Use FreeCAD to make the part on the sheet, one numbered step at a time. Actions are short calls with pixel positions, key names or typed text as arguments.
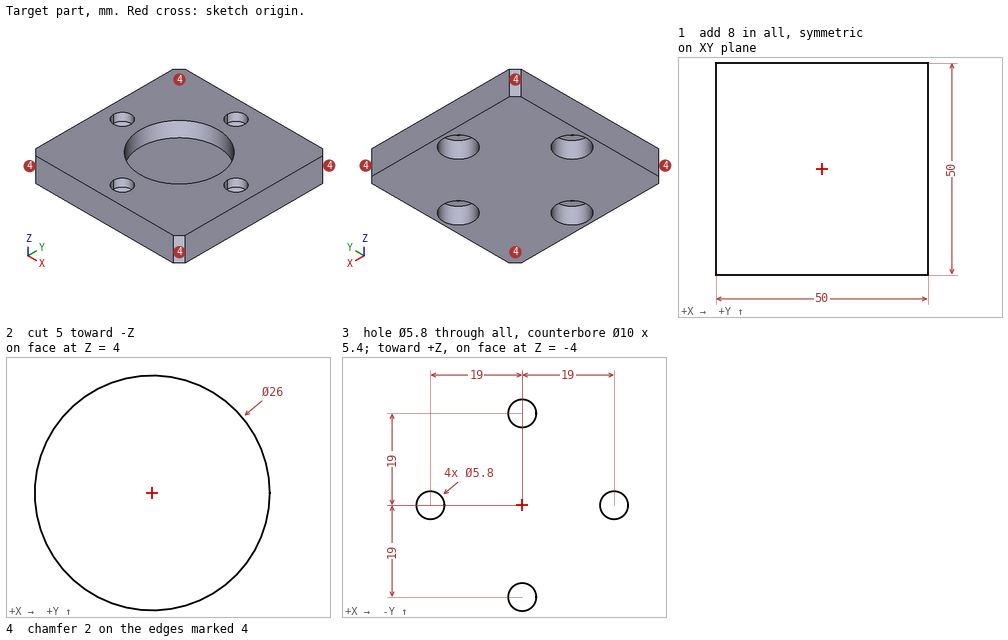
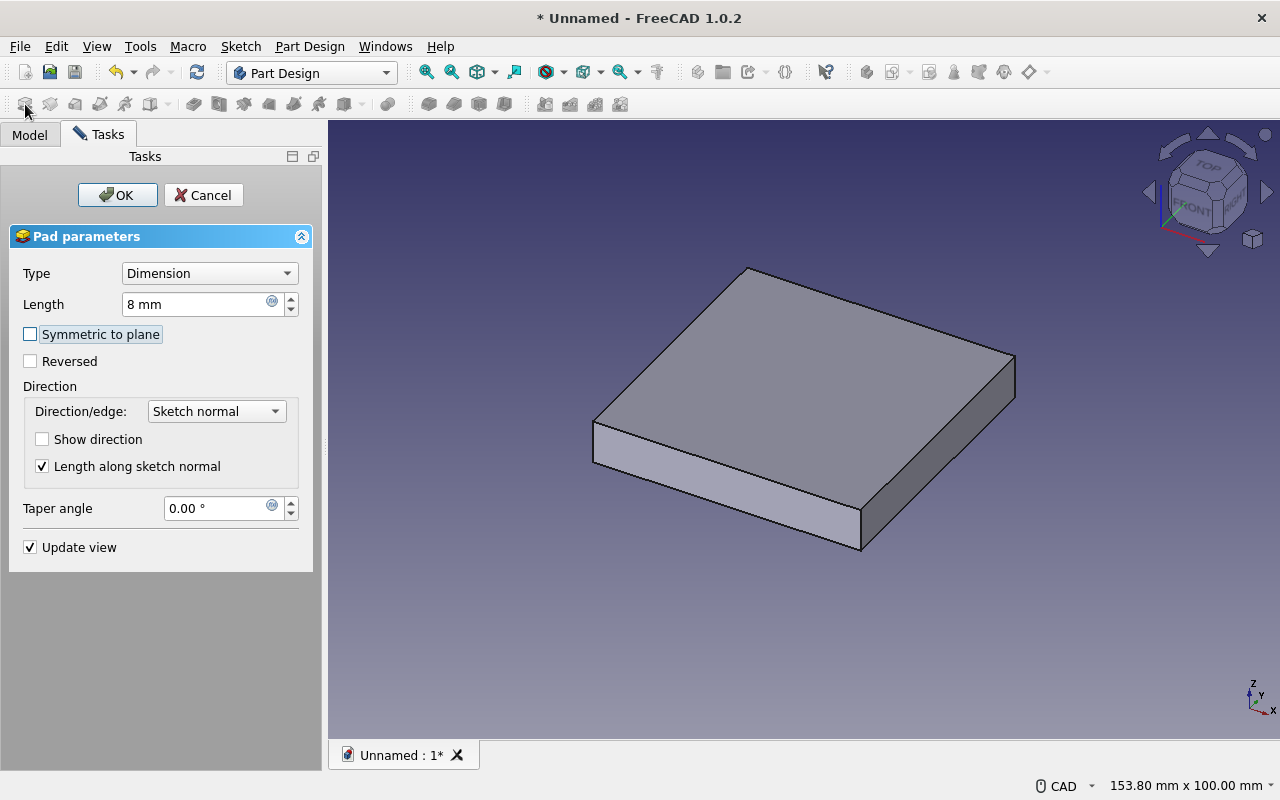
click(31, 334)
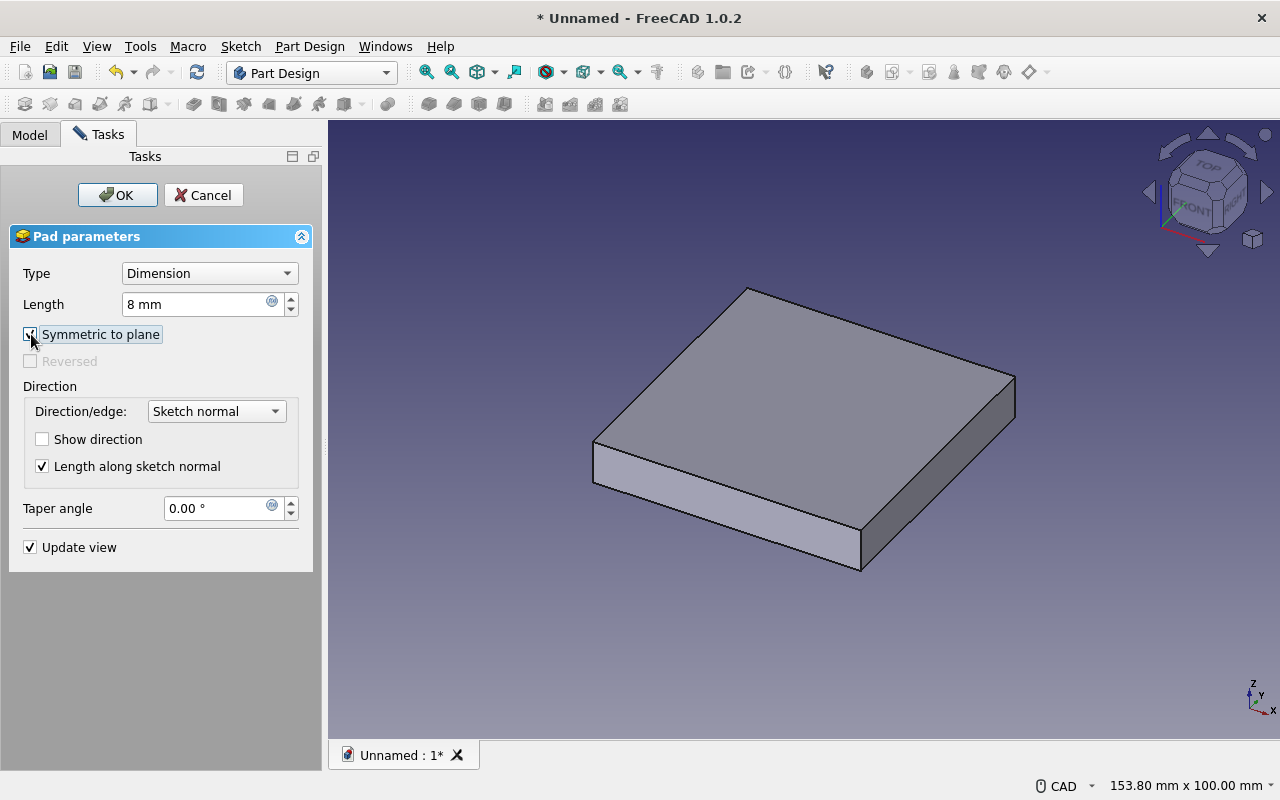
click(118, 195)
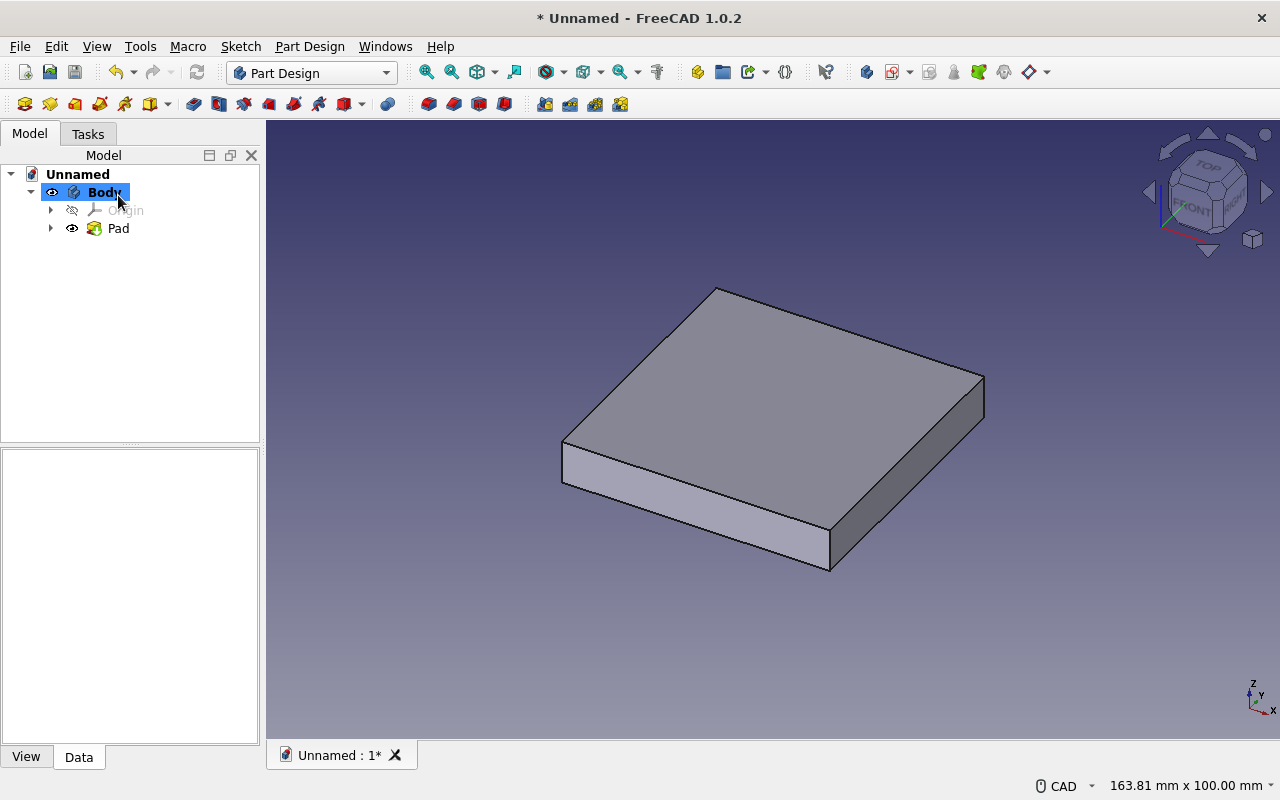
click(773, 408)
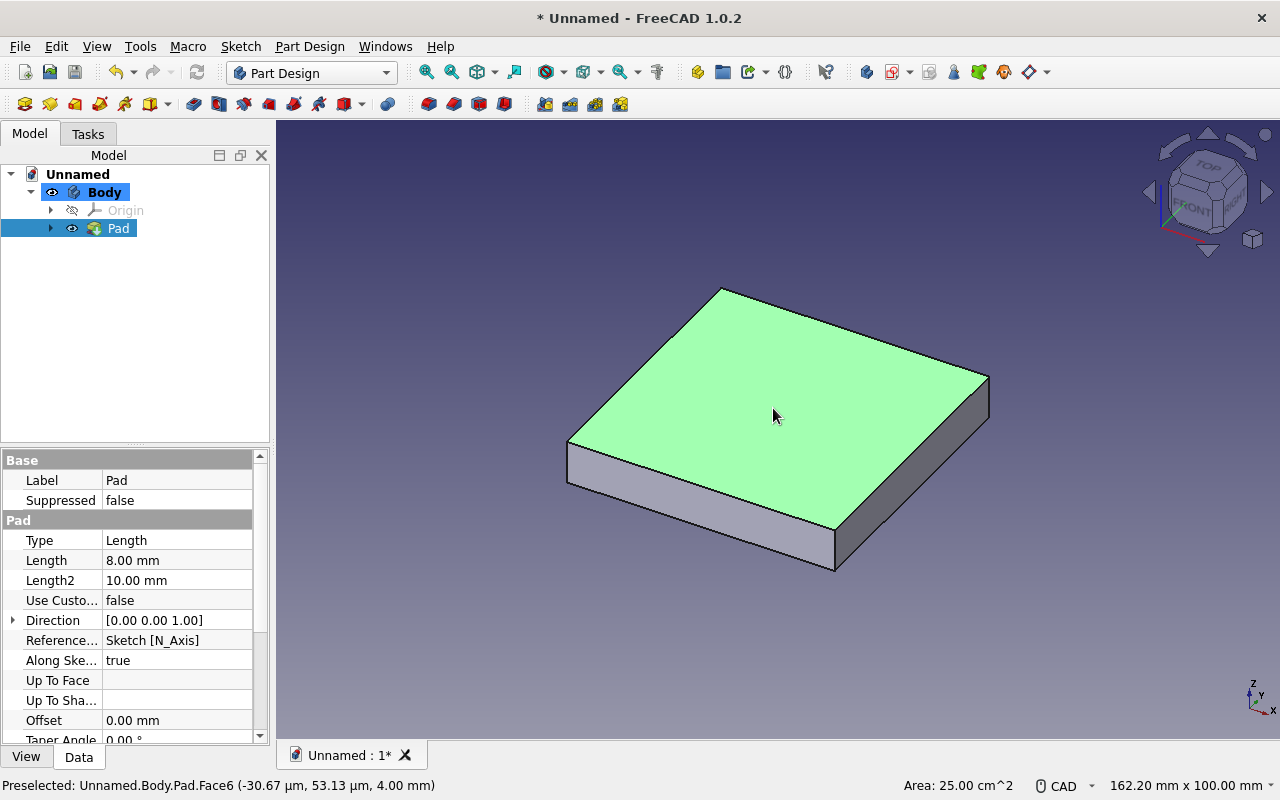
click(892, 72)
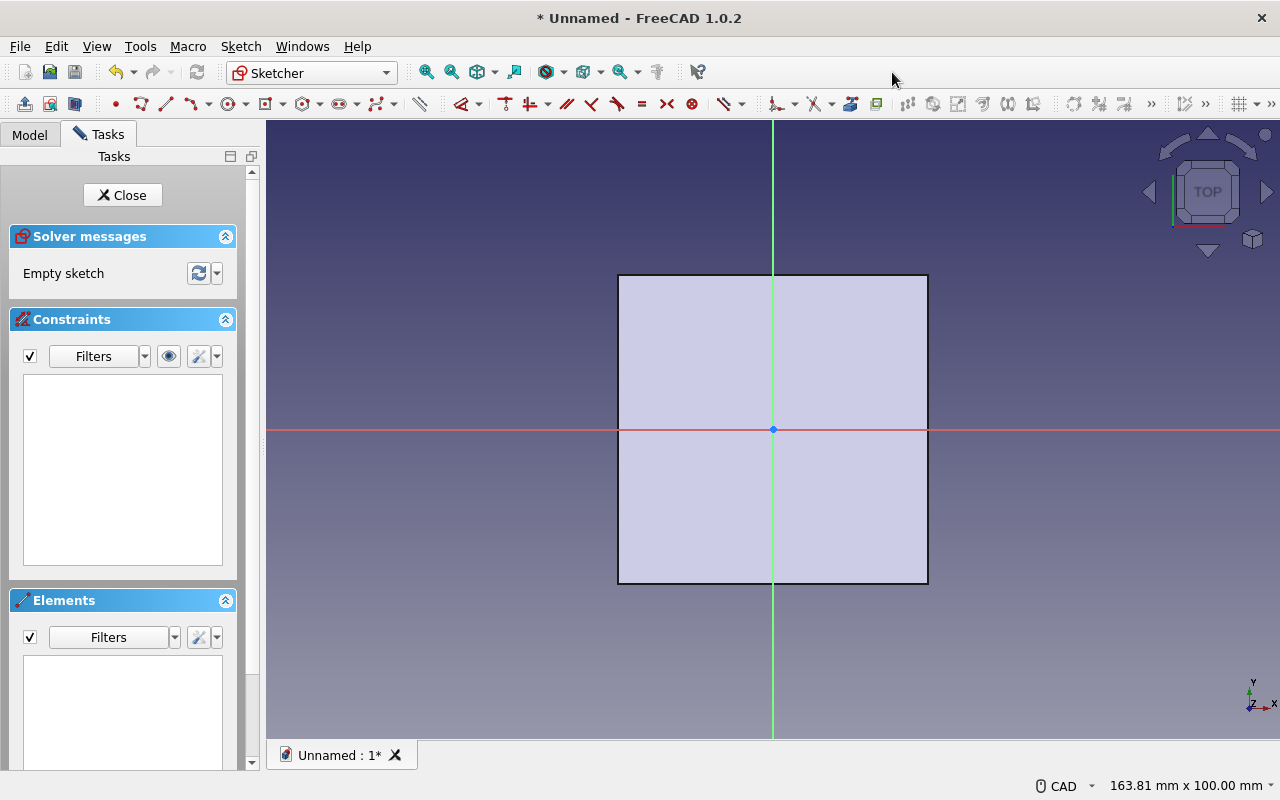
scroll(813, 429, up, 5)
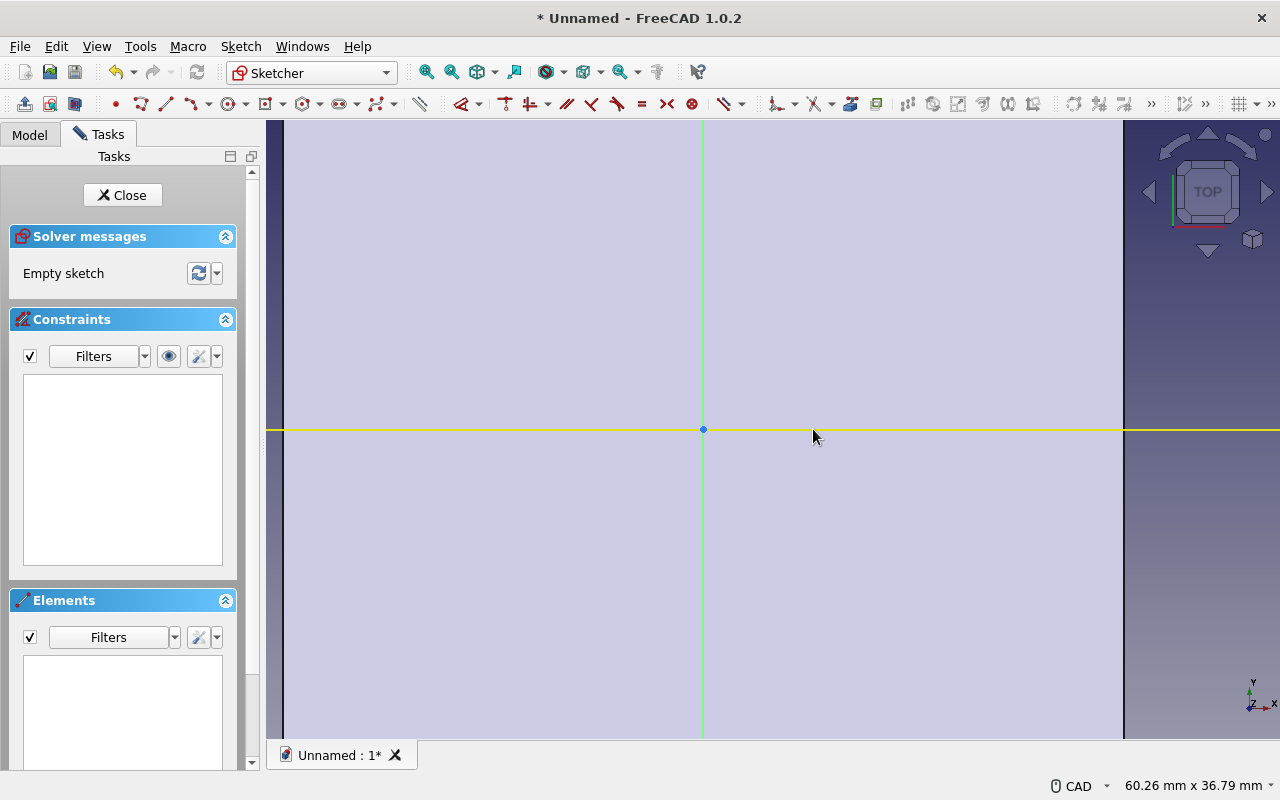
click(228, 104)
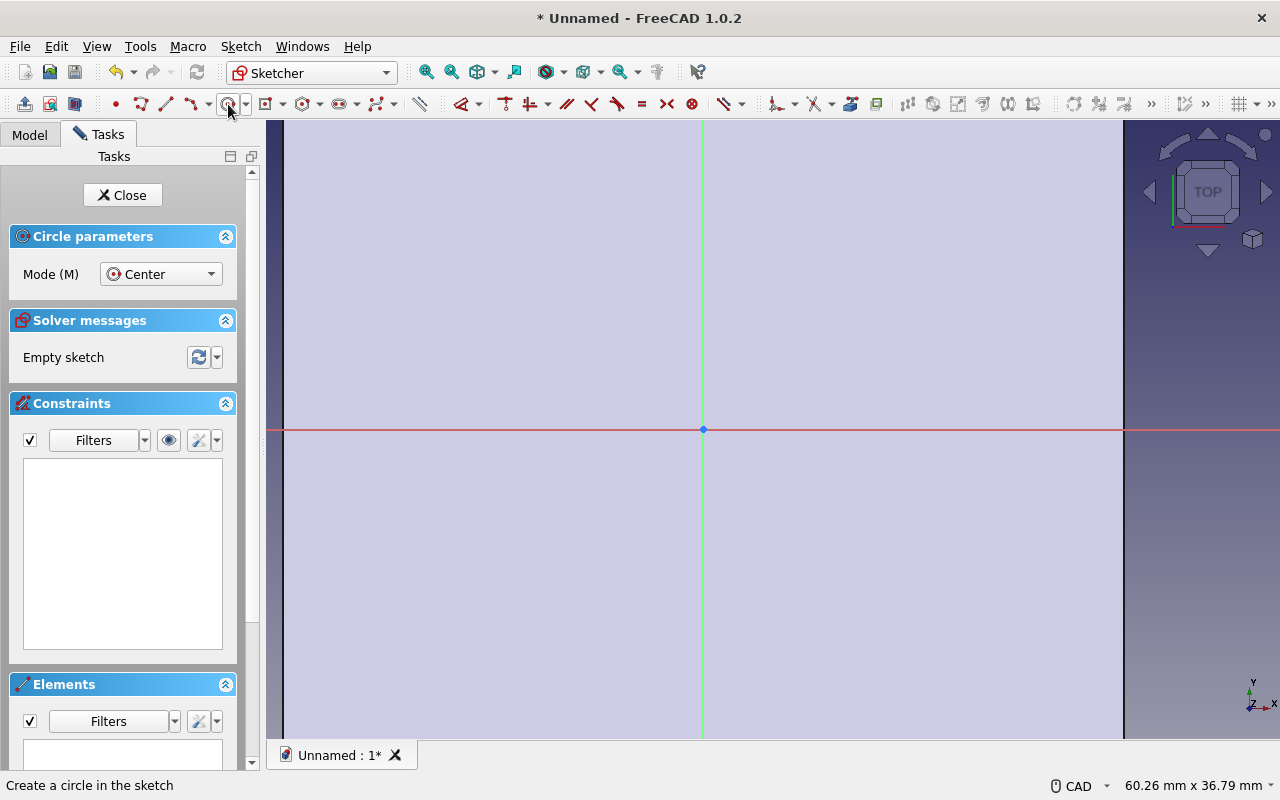
click(703, 430)
move(858, 275)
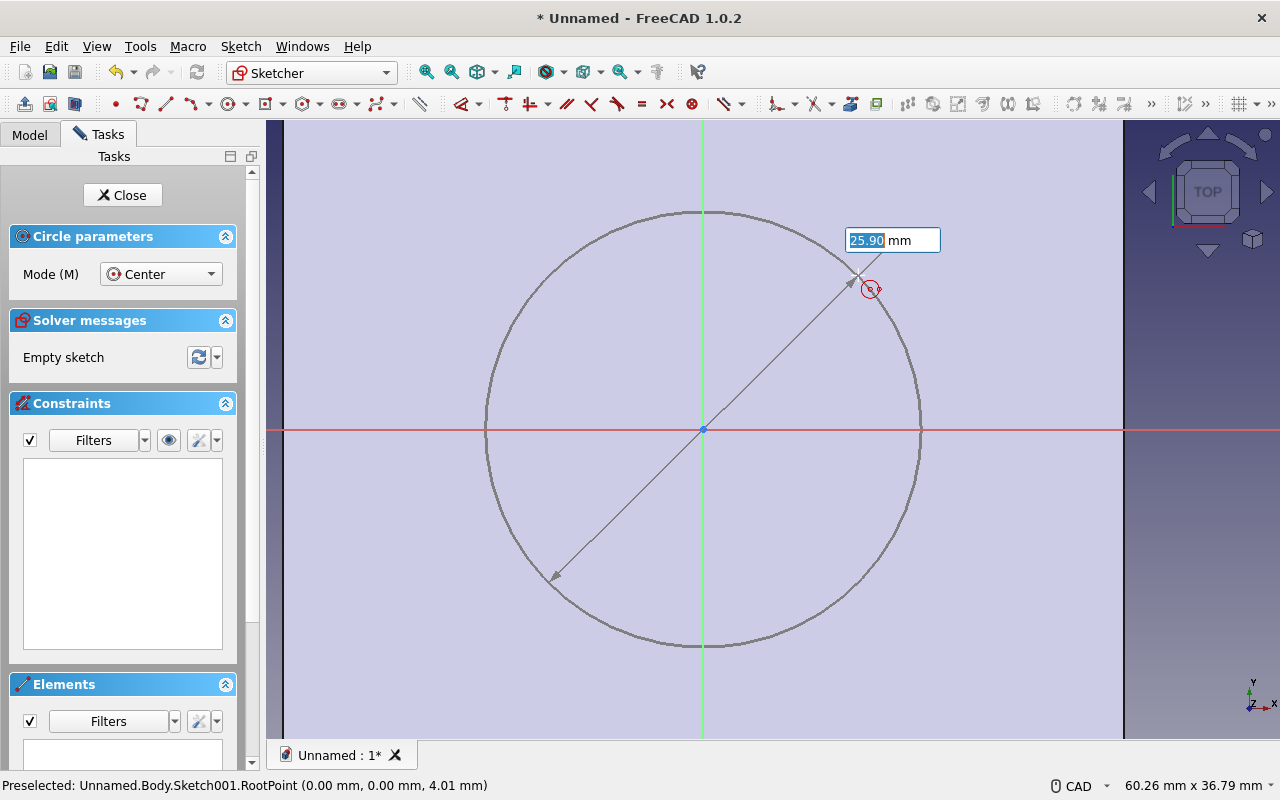
text(26)
key(Return)
key(Escape)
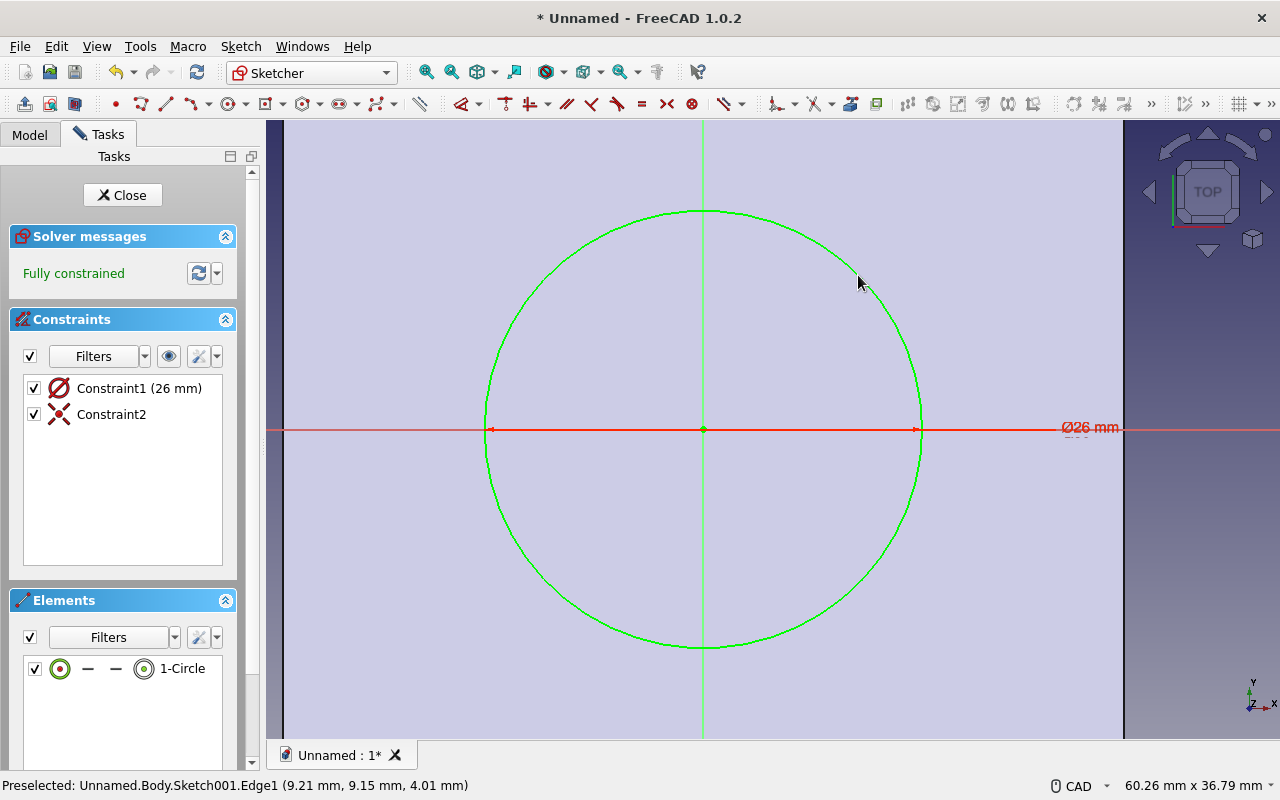
click(123, 195)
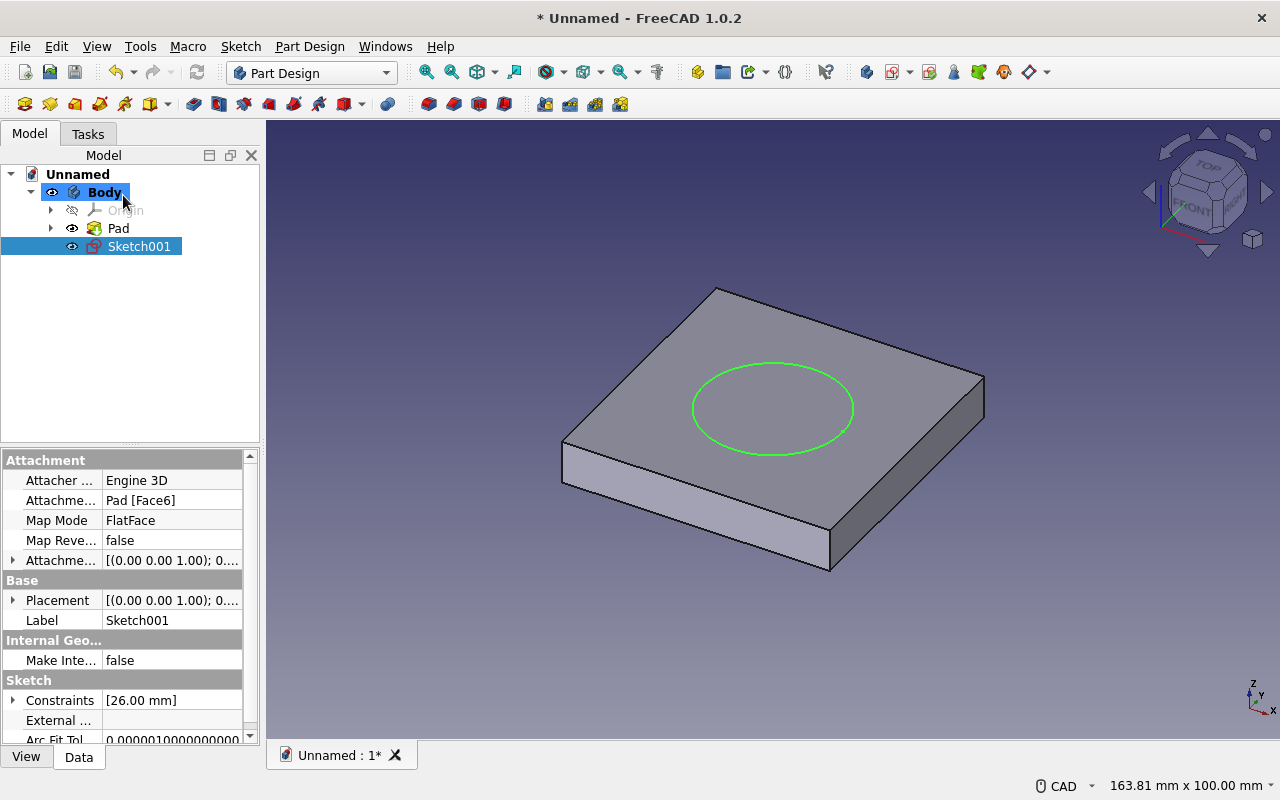
click(194, 104)